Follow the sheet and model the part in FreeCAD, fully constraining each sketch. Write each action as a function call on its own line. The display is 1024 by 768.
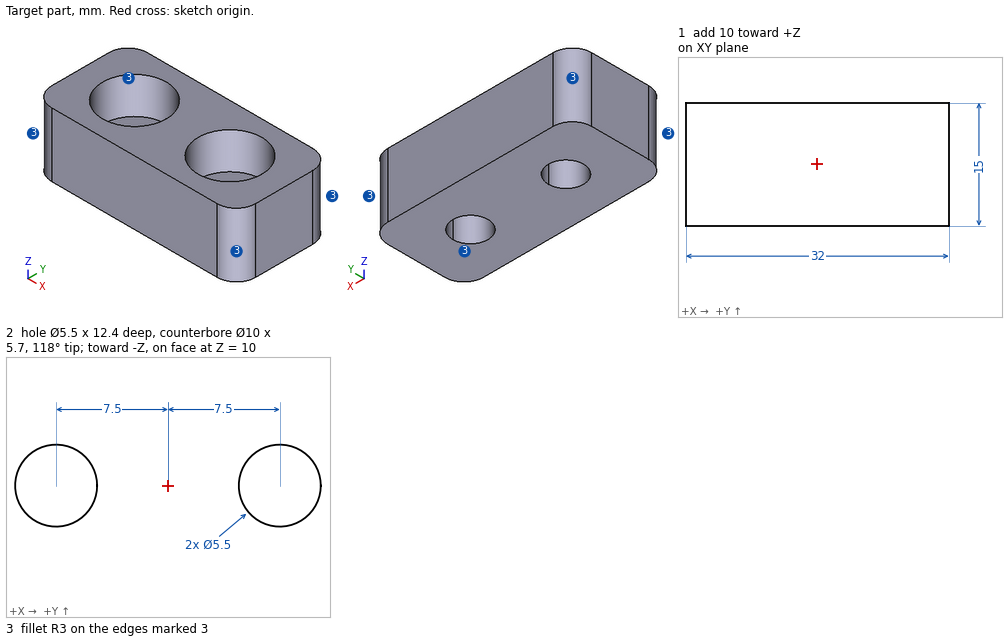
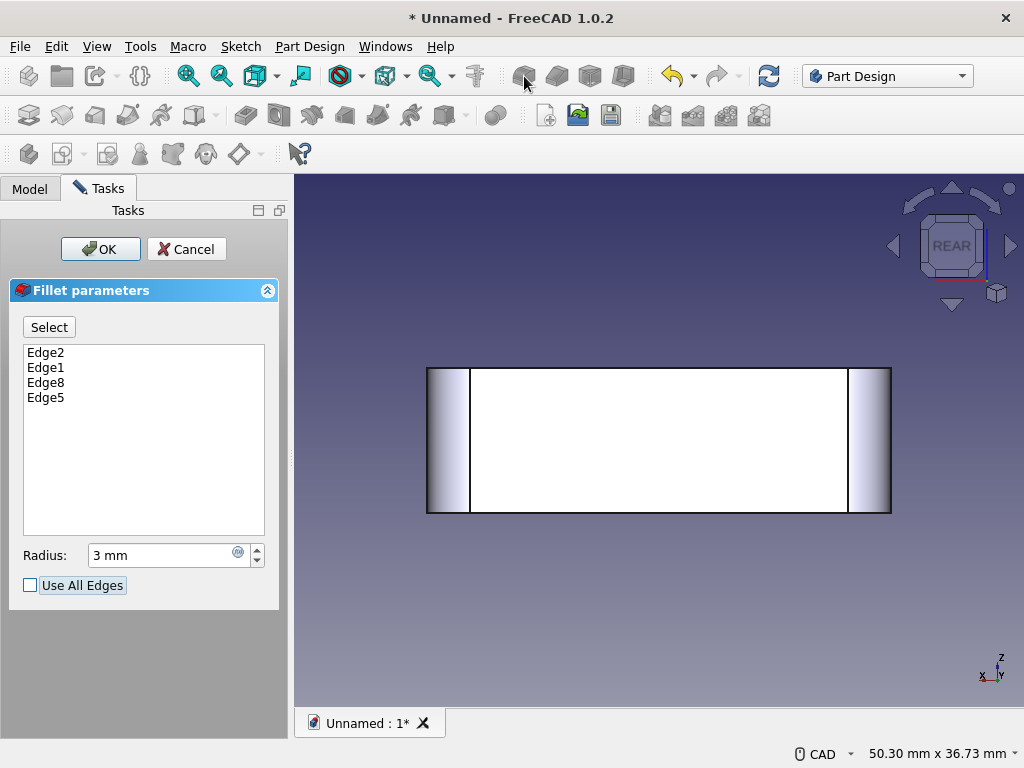
click(101, 249)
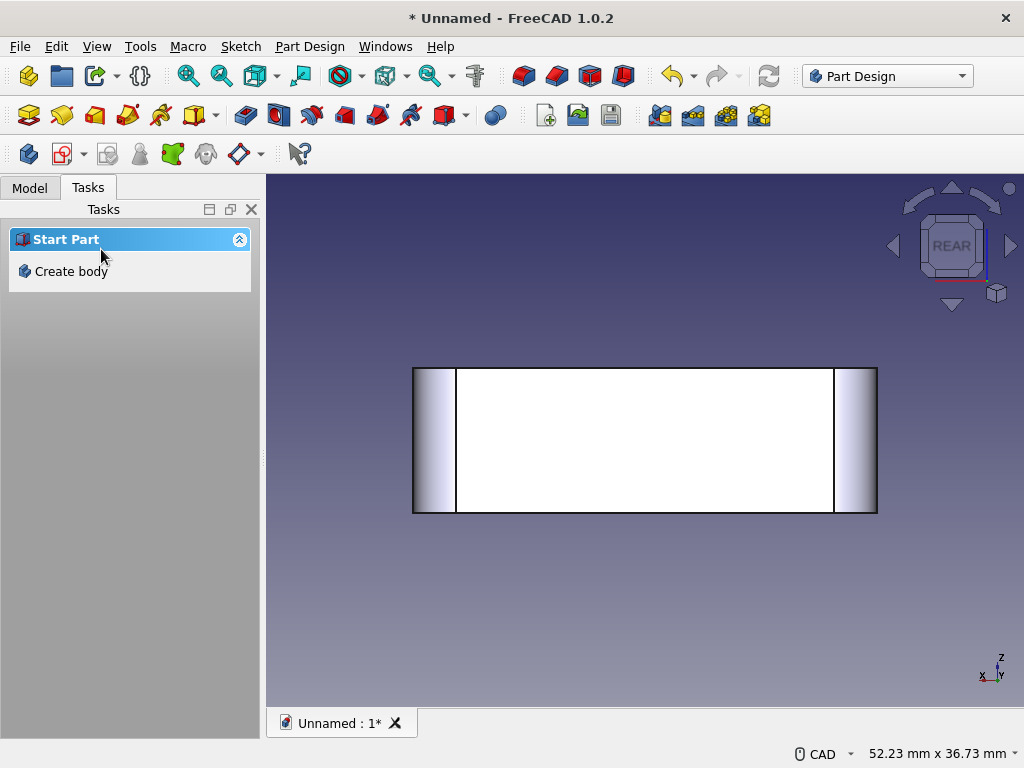
key(0)